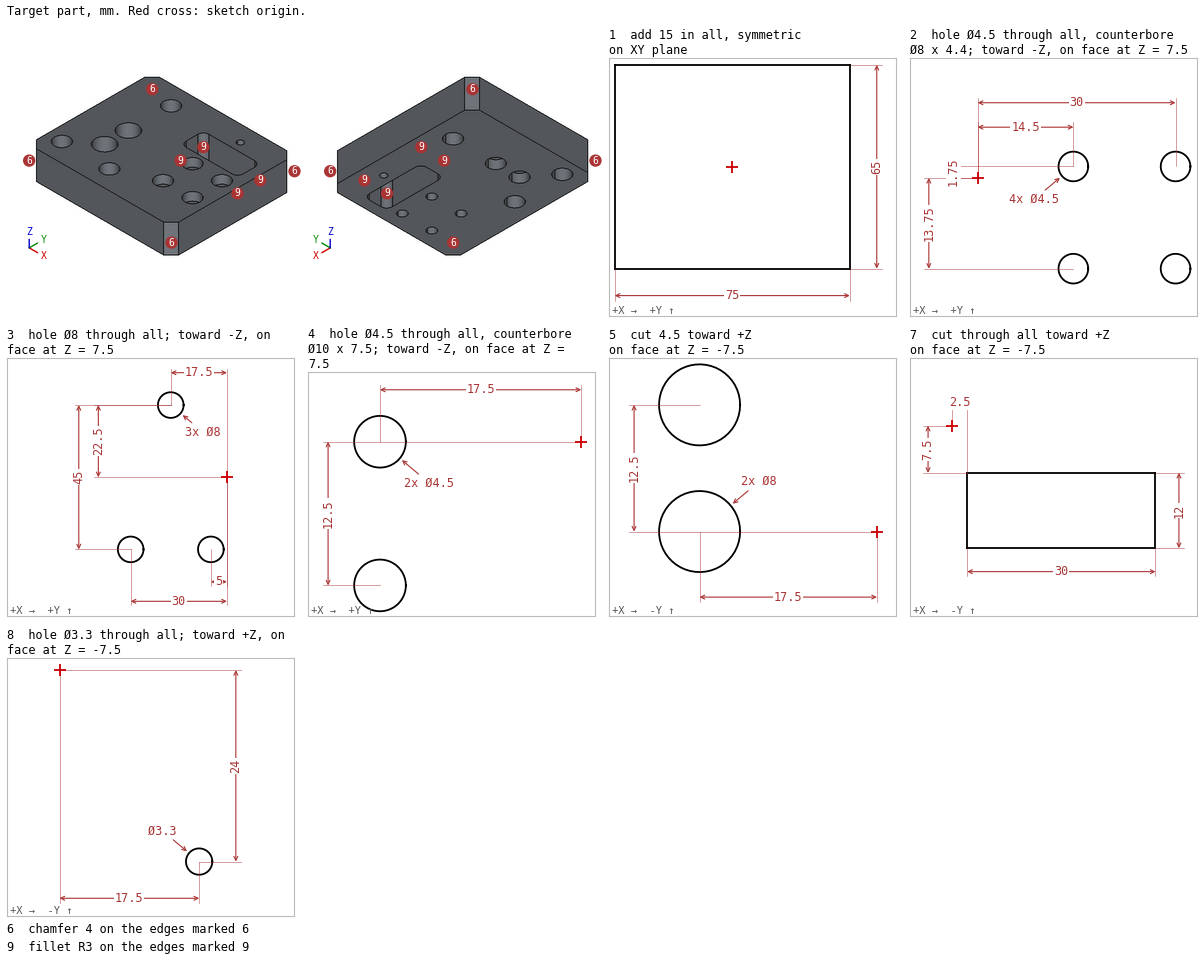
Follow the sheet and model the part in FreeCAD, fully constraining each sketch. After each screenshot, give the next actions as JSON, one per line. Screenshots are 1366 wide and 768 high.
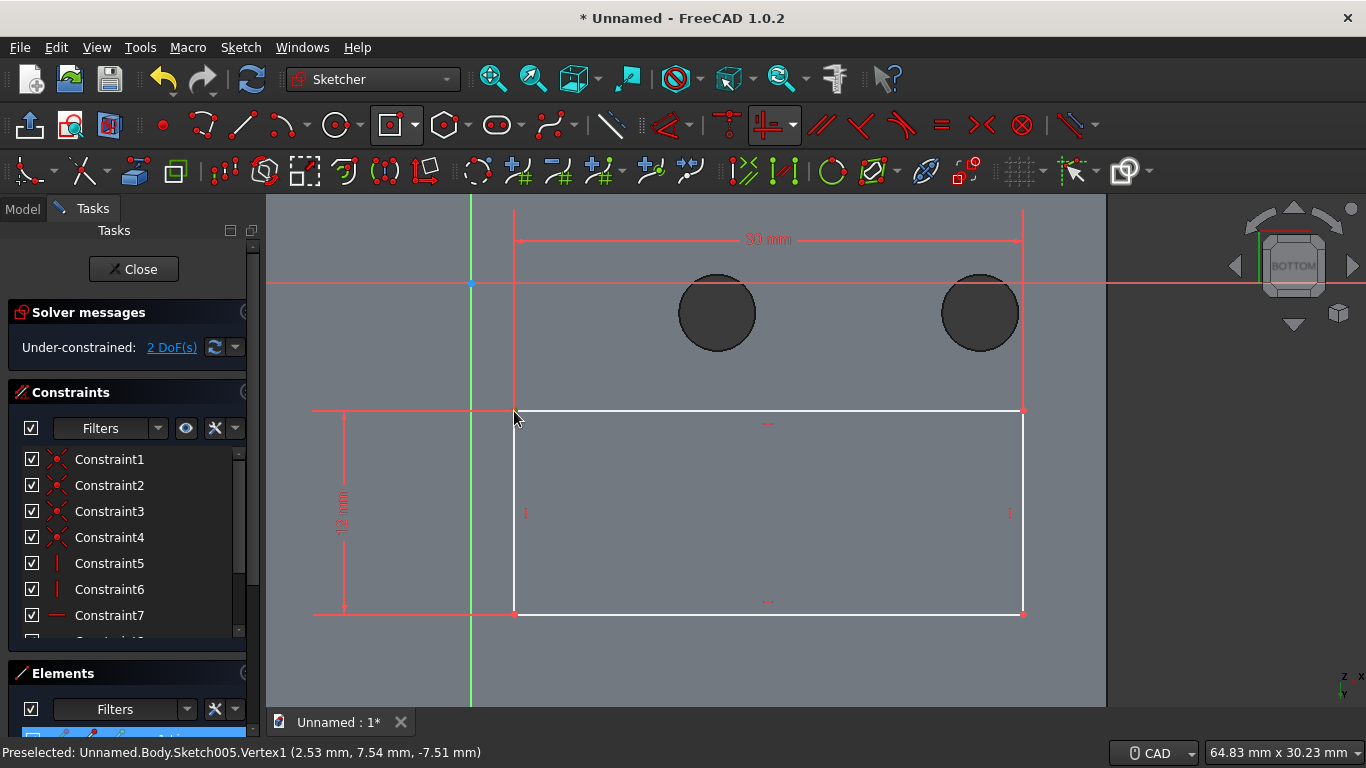
{"action": "key", "text": "l"}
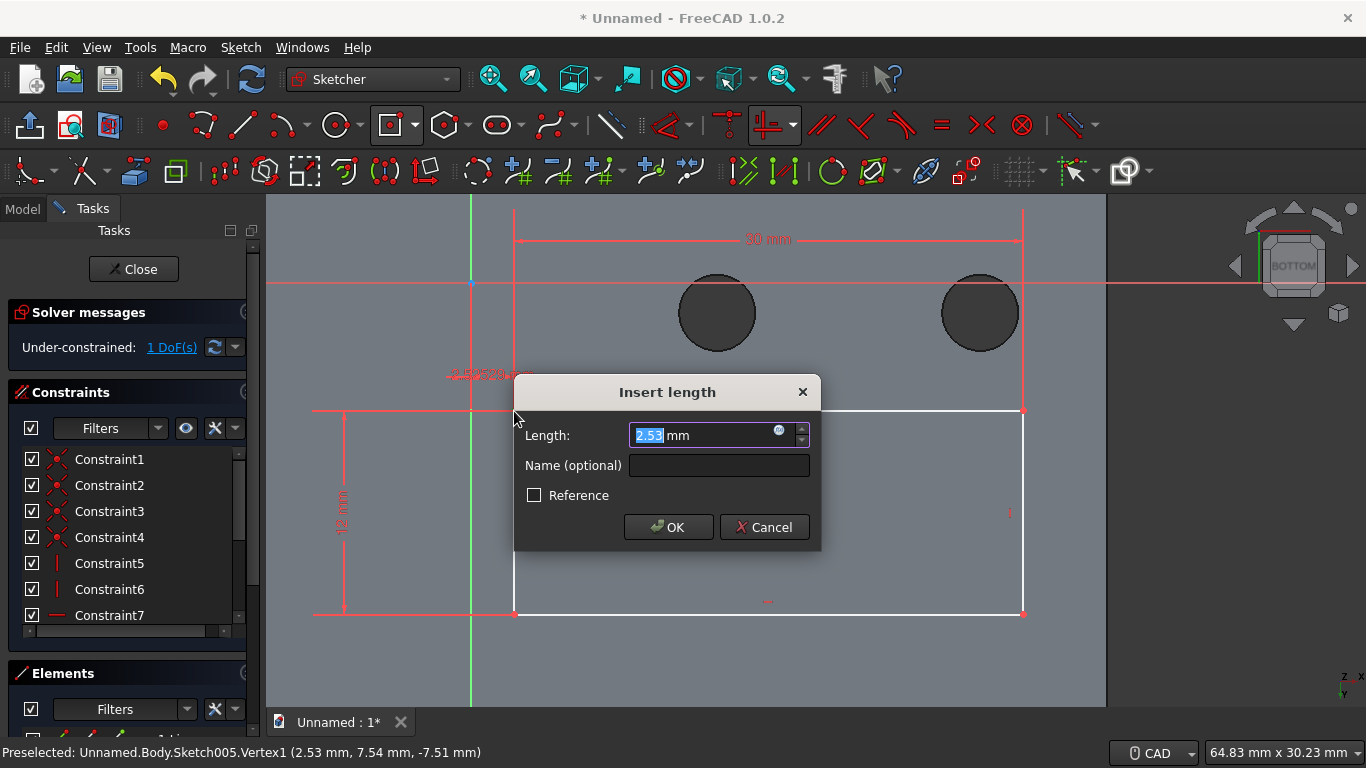
{"action": "type", "text": "2.5"}
{"action": "key", "text": "Return"}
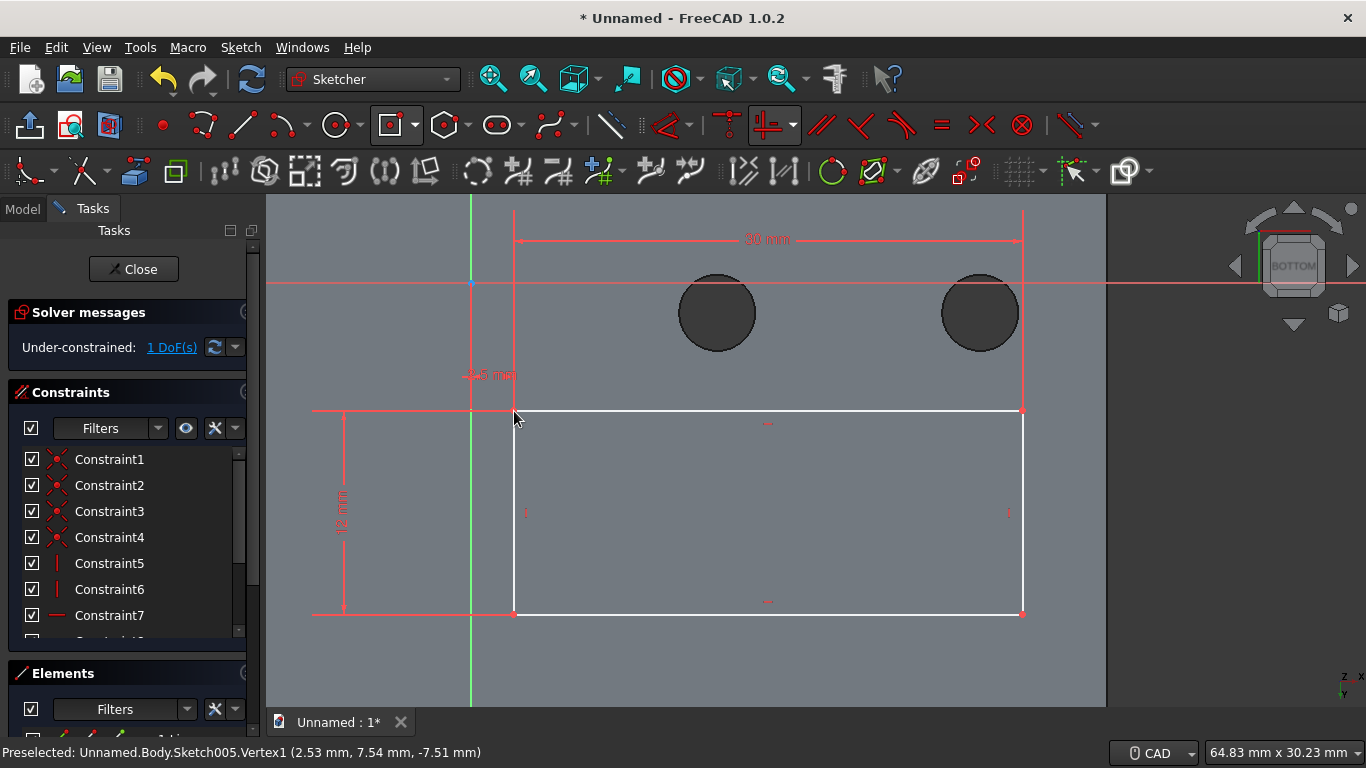
{"action": "left_click", "coordinate": [514, 411]}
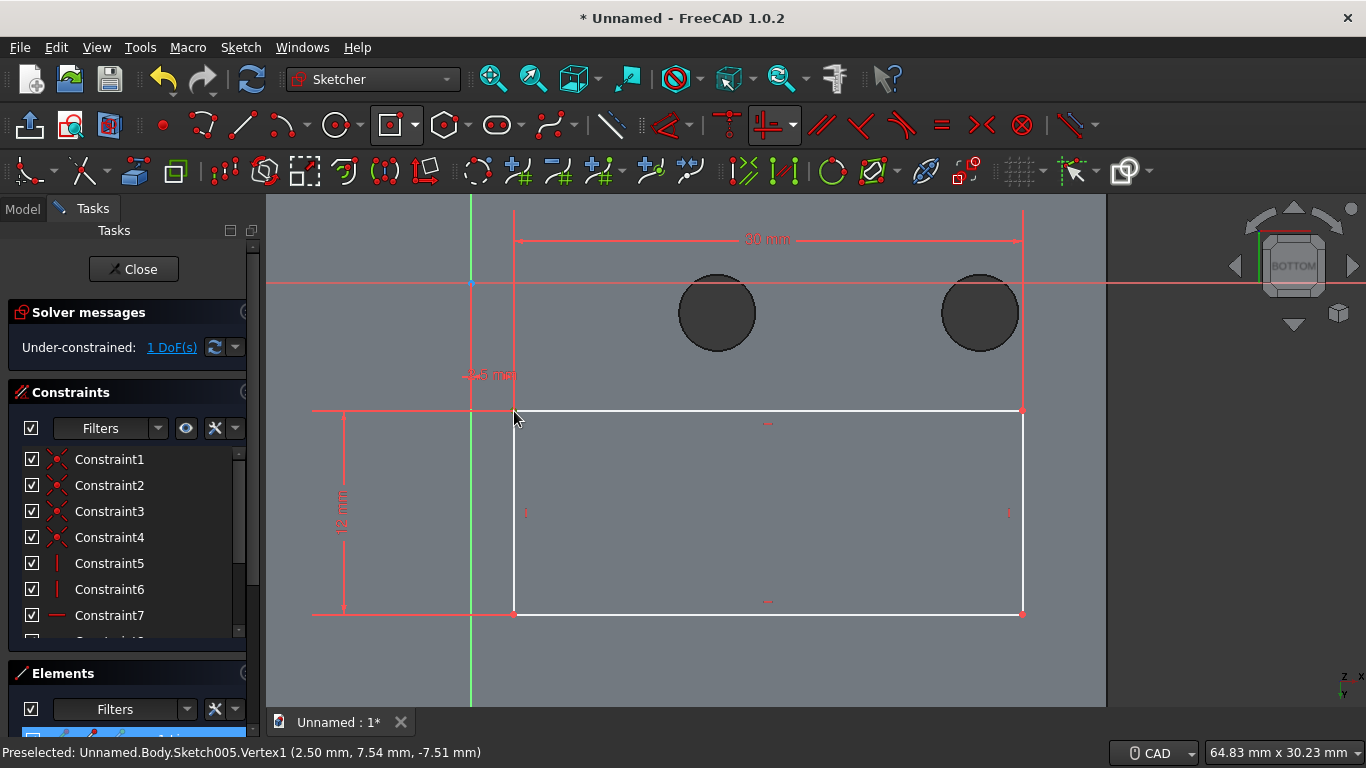
{"action": "left_click", "coordinate": [692, 126]}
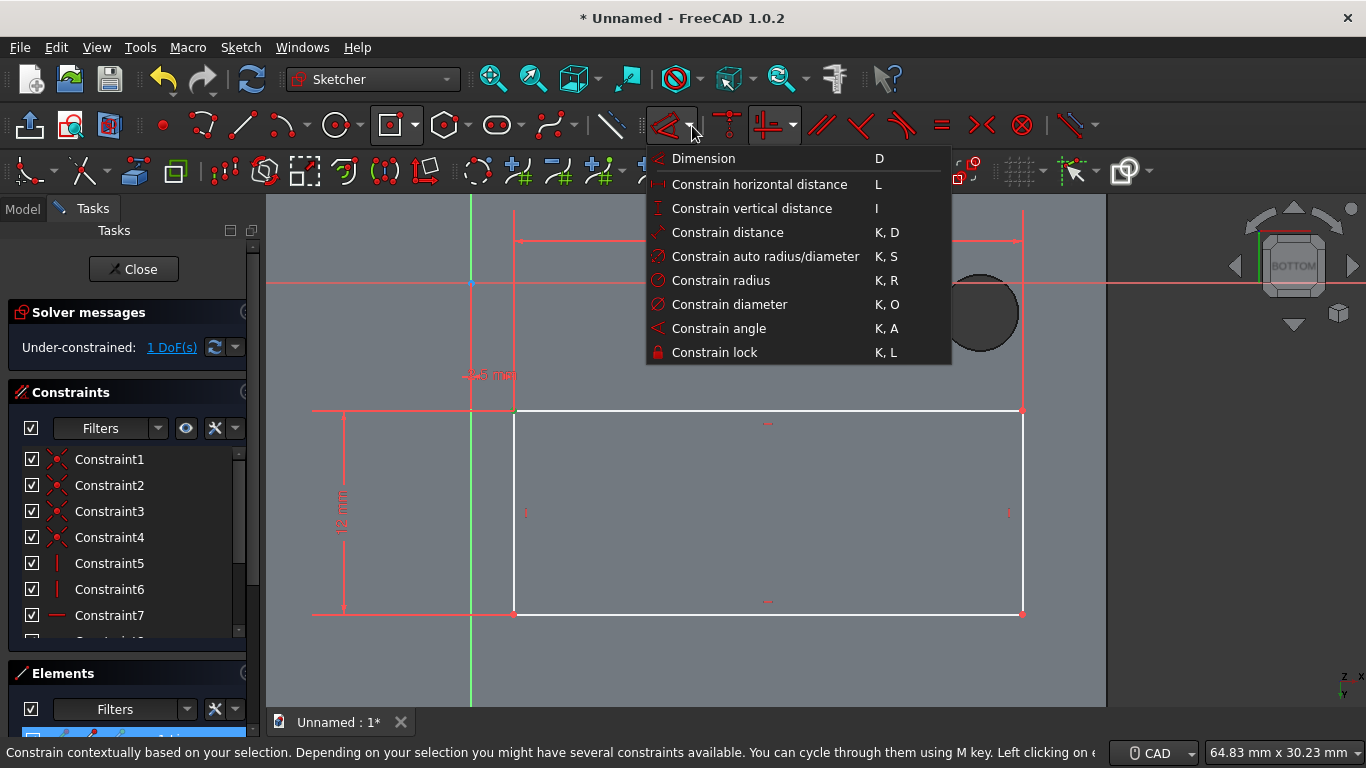
{"action": "left_click", "coordinate": [799, 208]}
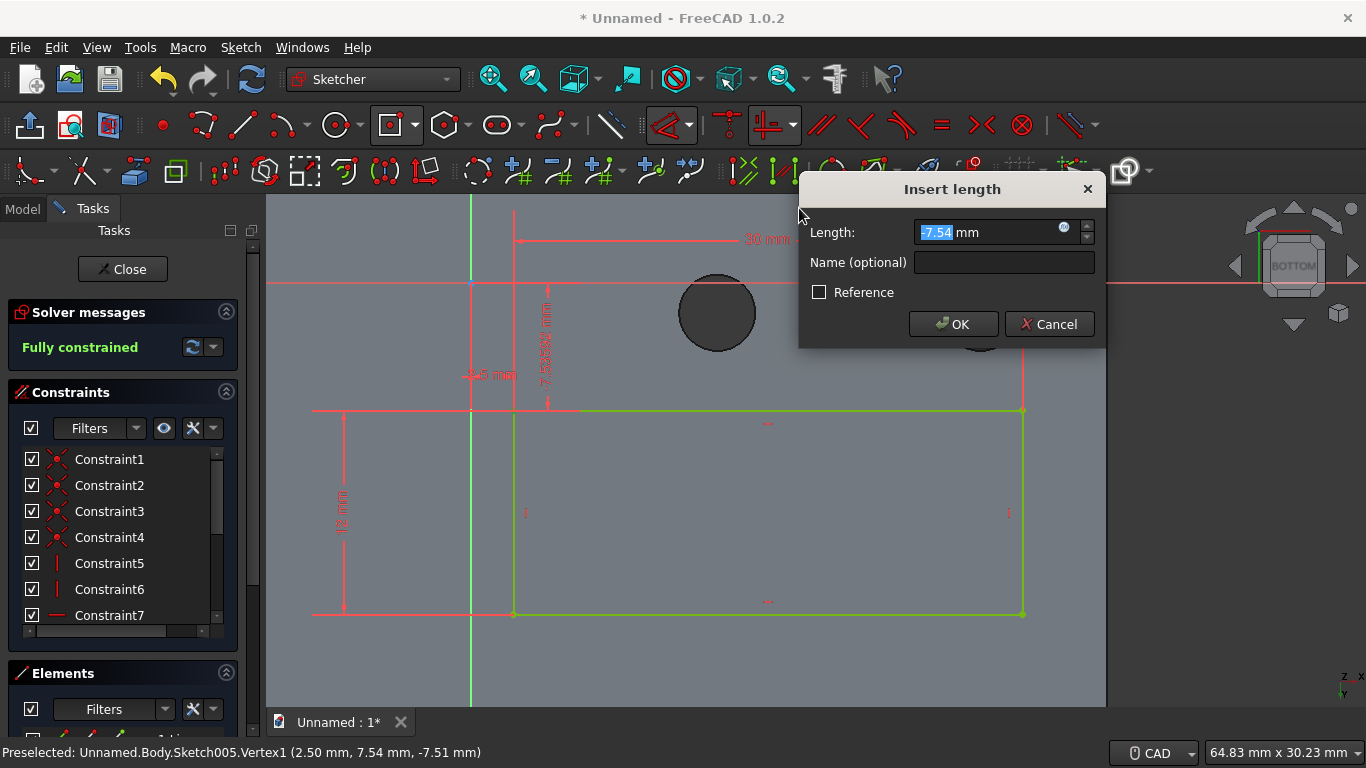
{"action": "type", "text": "-7.5"}
{"action": "key", "text": "Return"}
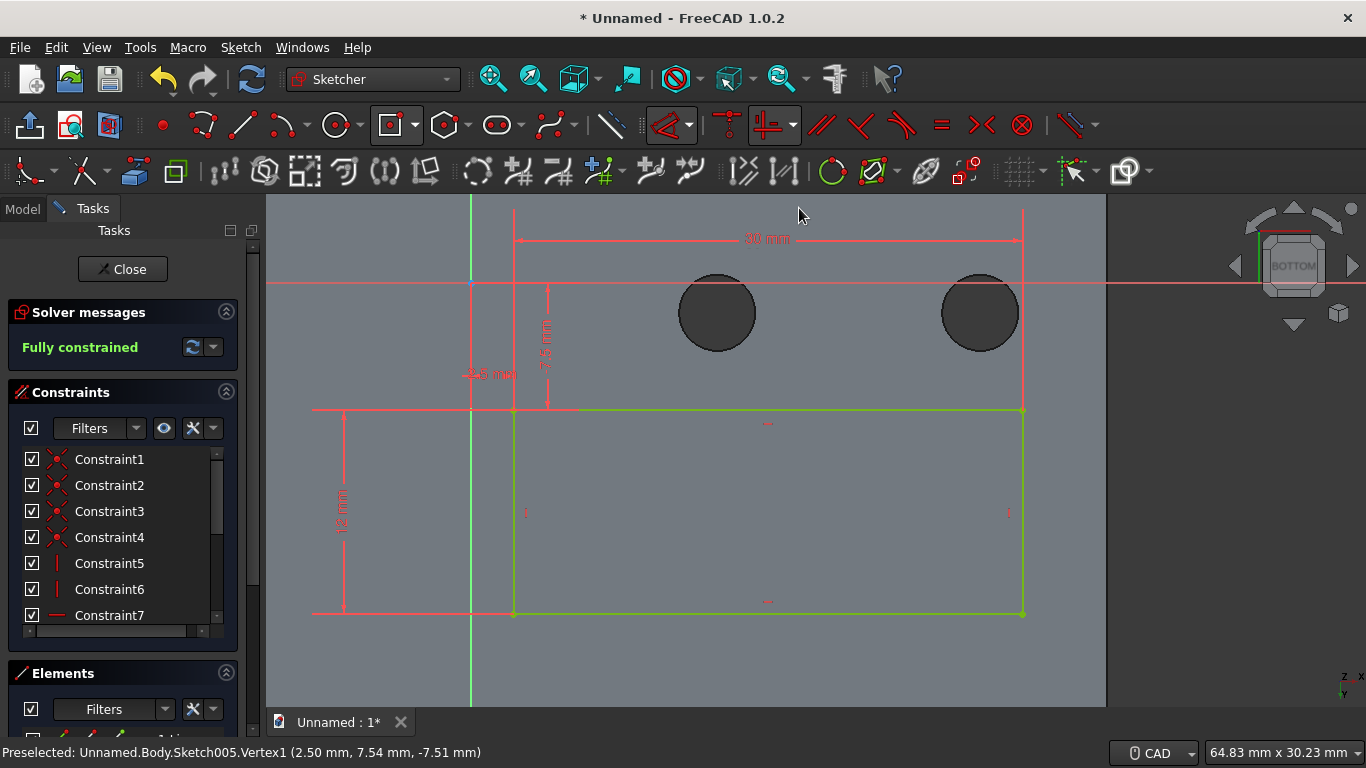
{"action": "left_click", "coordinate": [123, 269]}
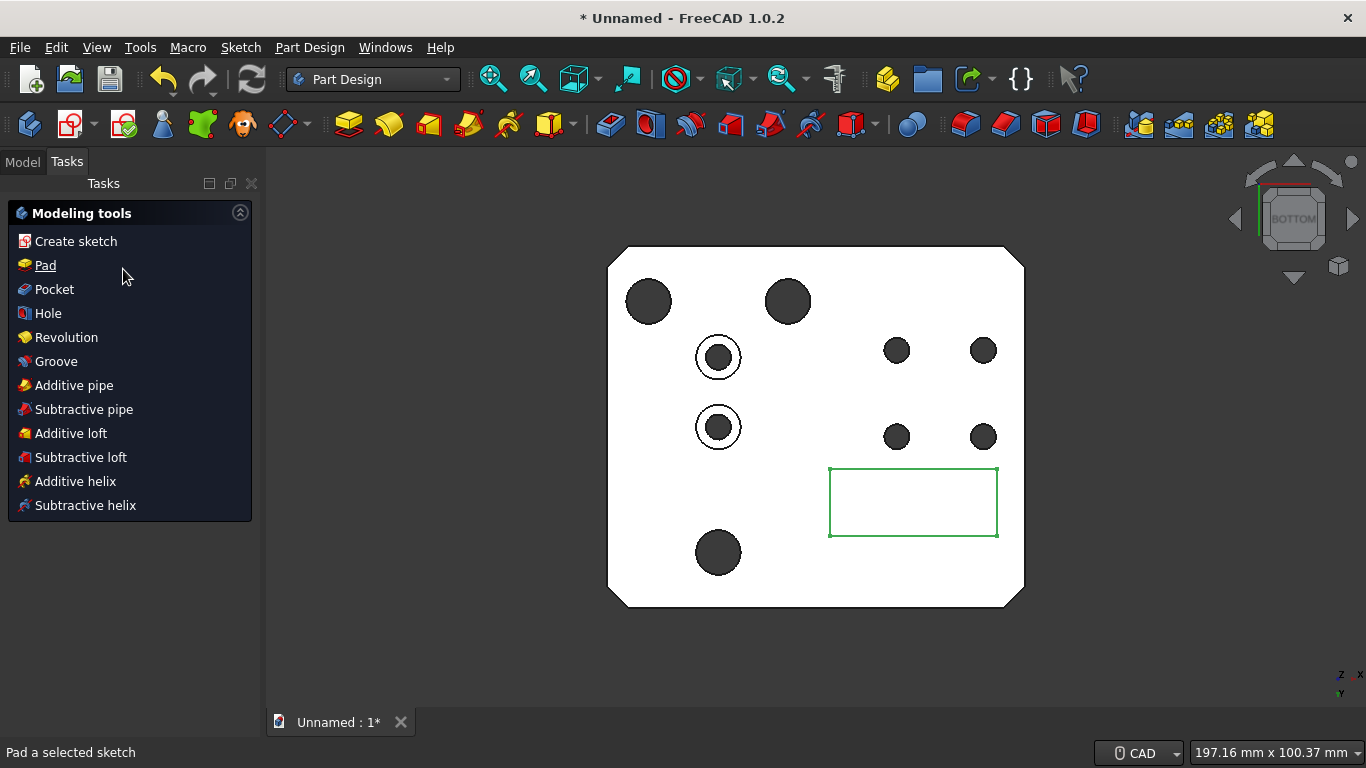
{"action": "left_click", "coordinate": [612, 124]}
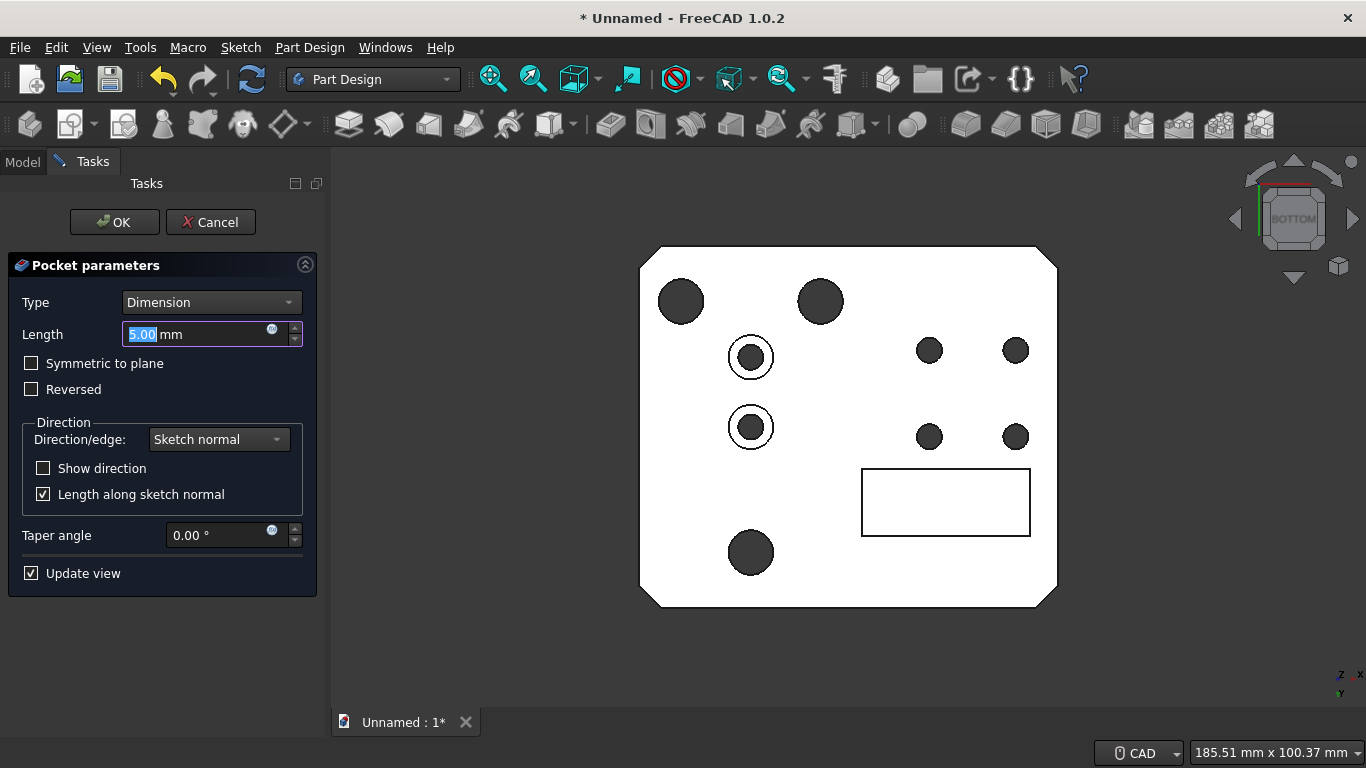
{"action": "left_click", "coordinate": [212, 302]}